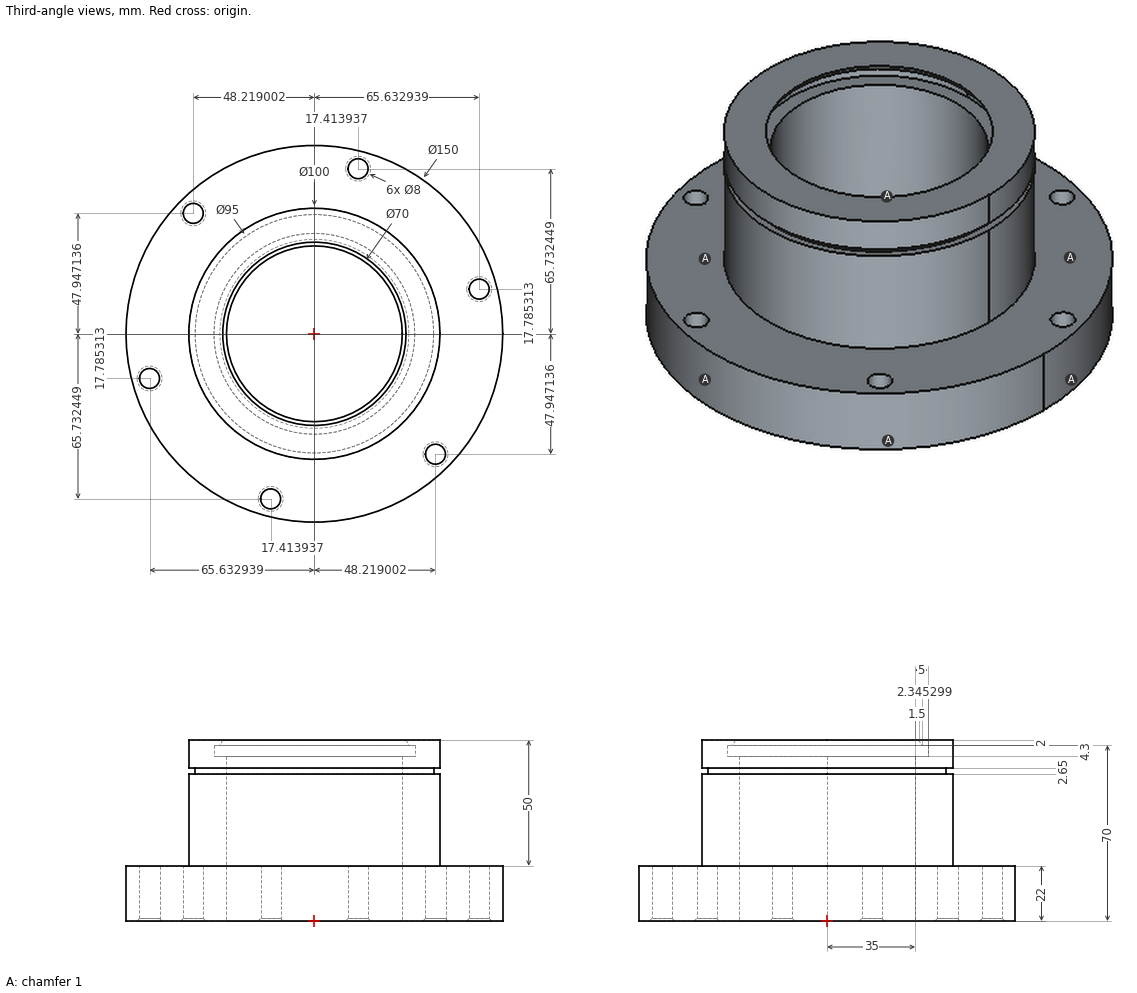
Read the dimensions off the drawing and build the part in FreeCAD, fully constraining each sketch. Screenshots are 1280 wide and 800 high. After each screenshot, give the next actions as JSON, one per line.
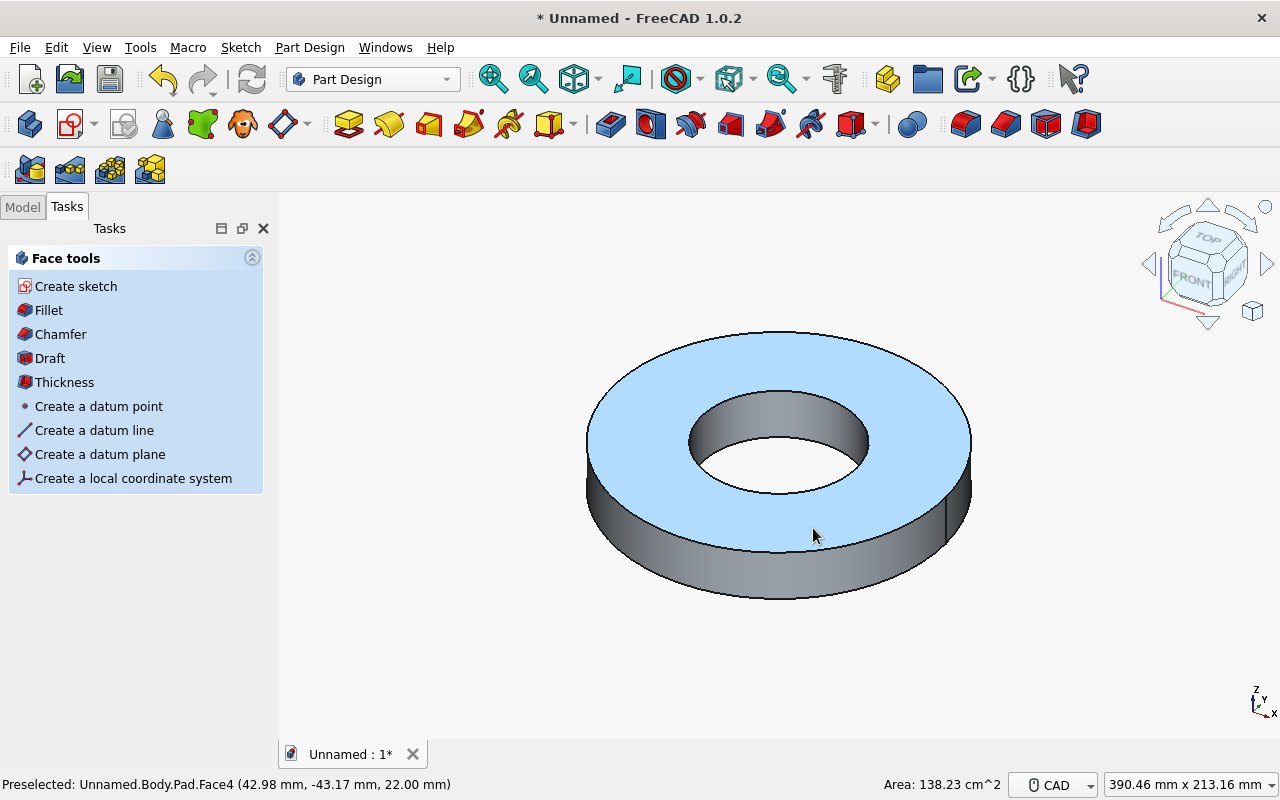
{"action": "left_click", "coordinate": [70, 124]}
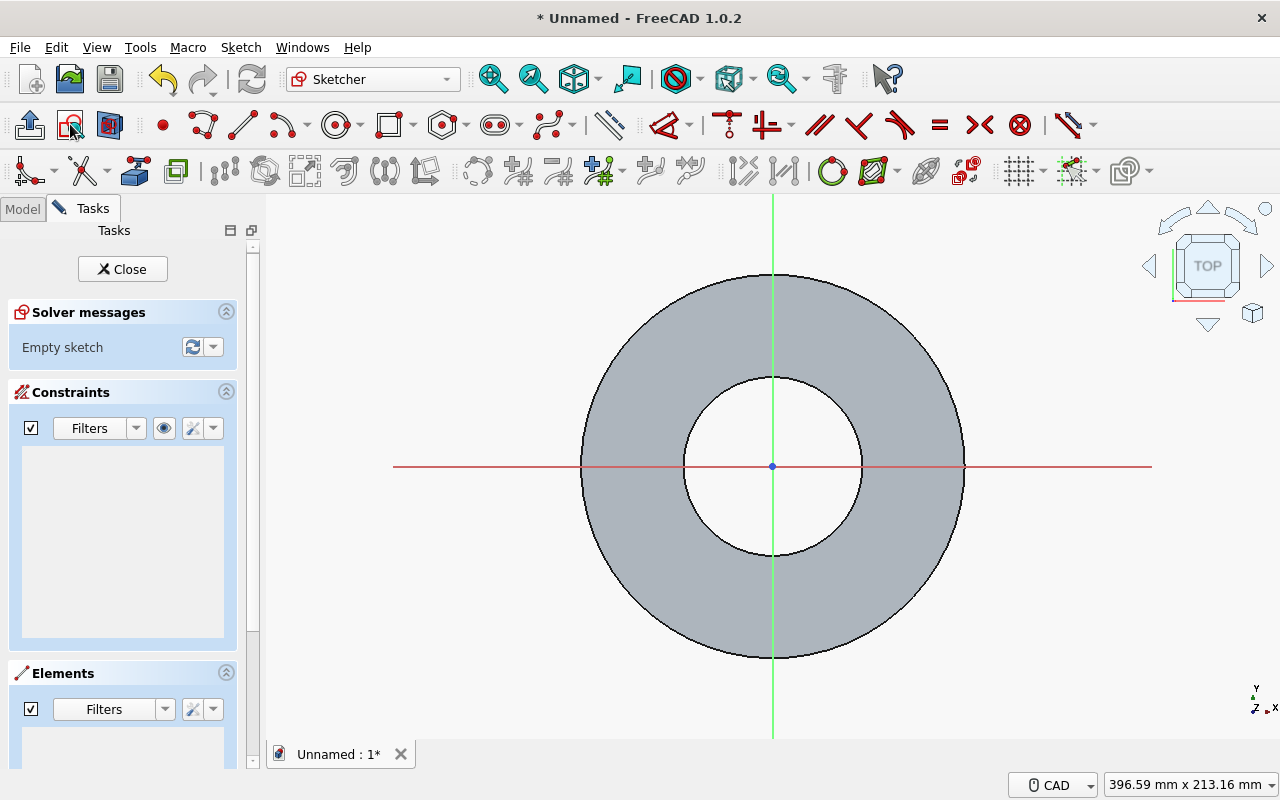
{"action": "left_click", "coordinate": [336, 126]}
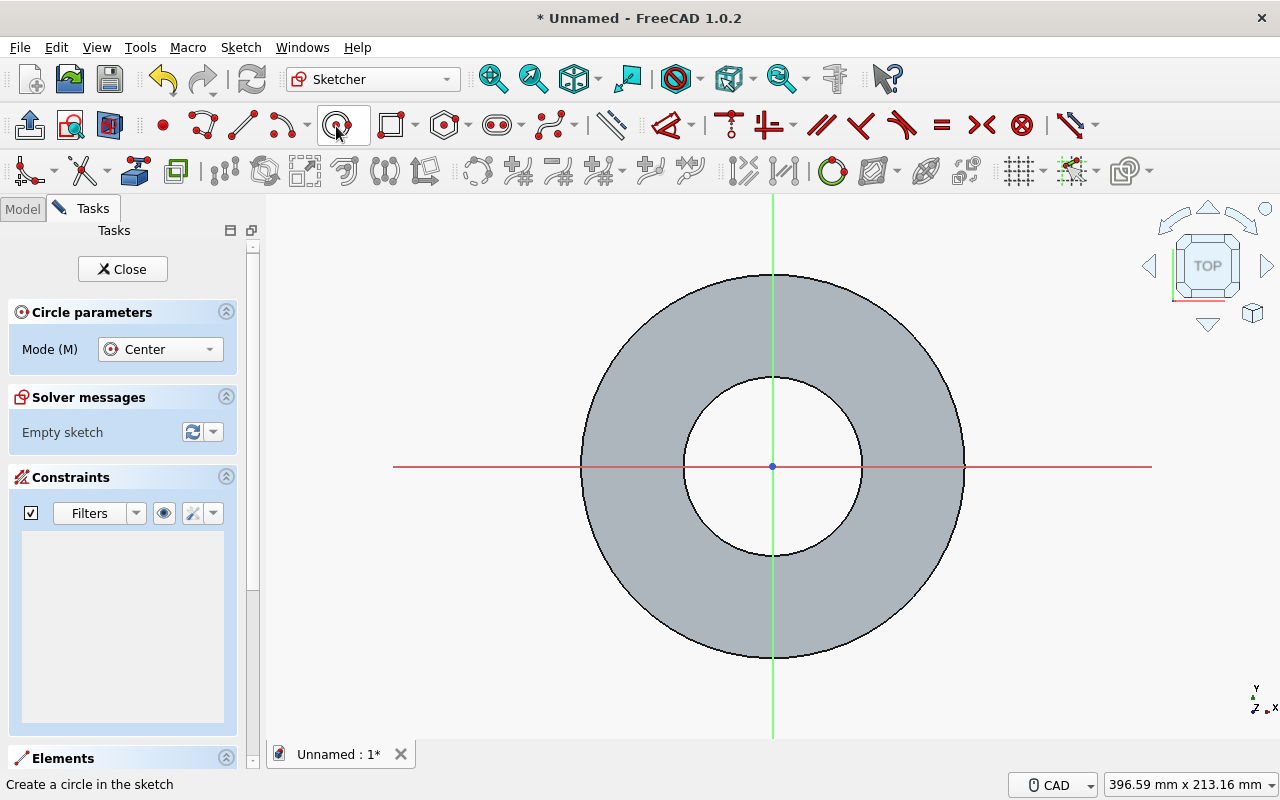
{"action": "left_click", "coordinate": [773, 466]}
{"action": "left_click", "coordinate": [863, 376]}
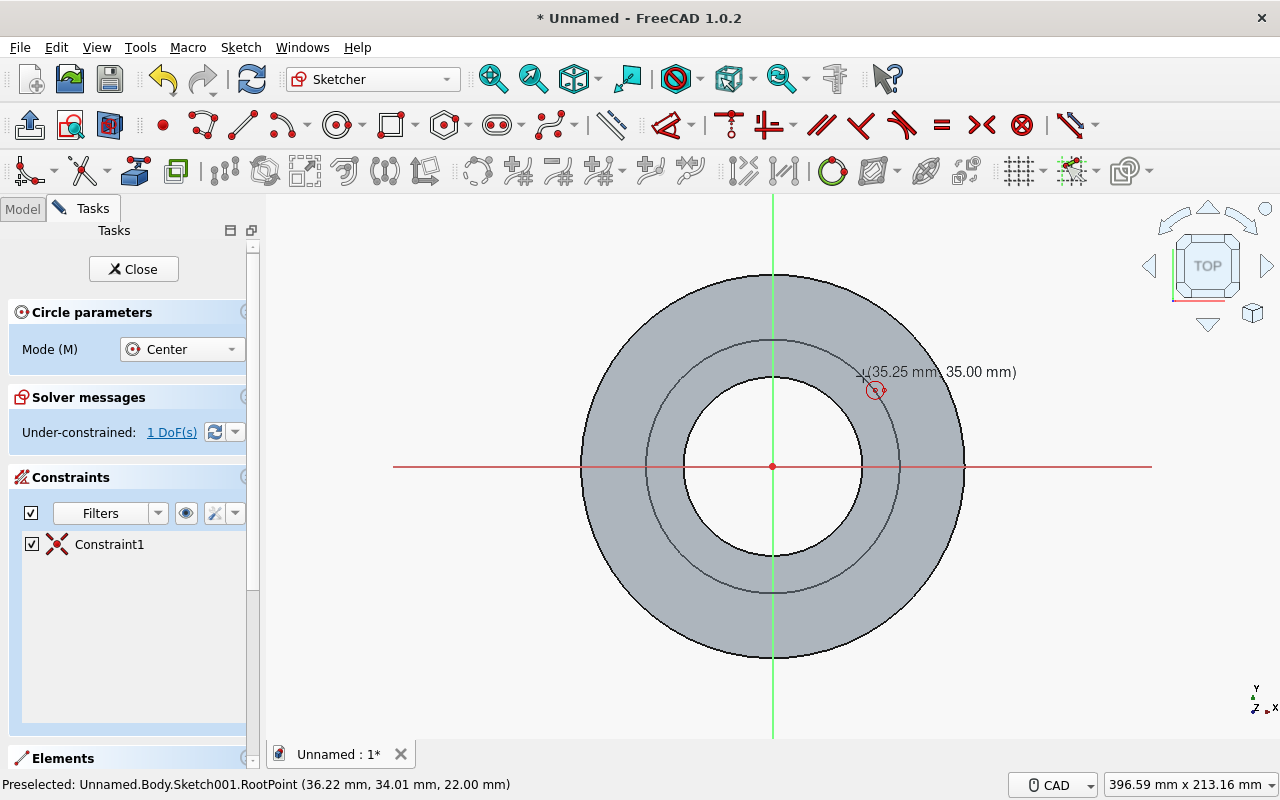
{"action": "left_click", "coordinate": [773, 466]}
{"action": "left_click", "coordinate": [836, 403]}
{"action": "key", "text": "Escape"}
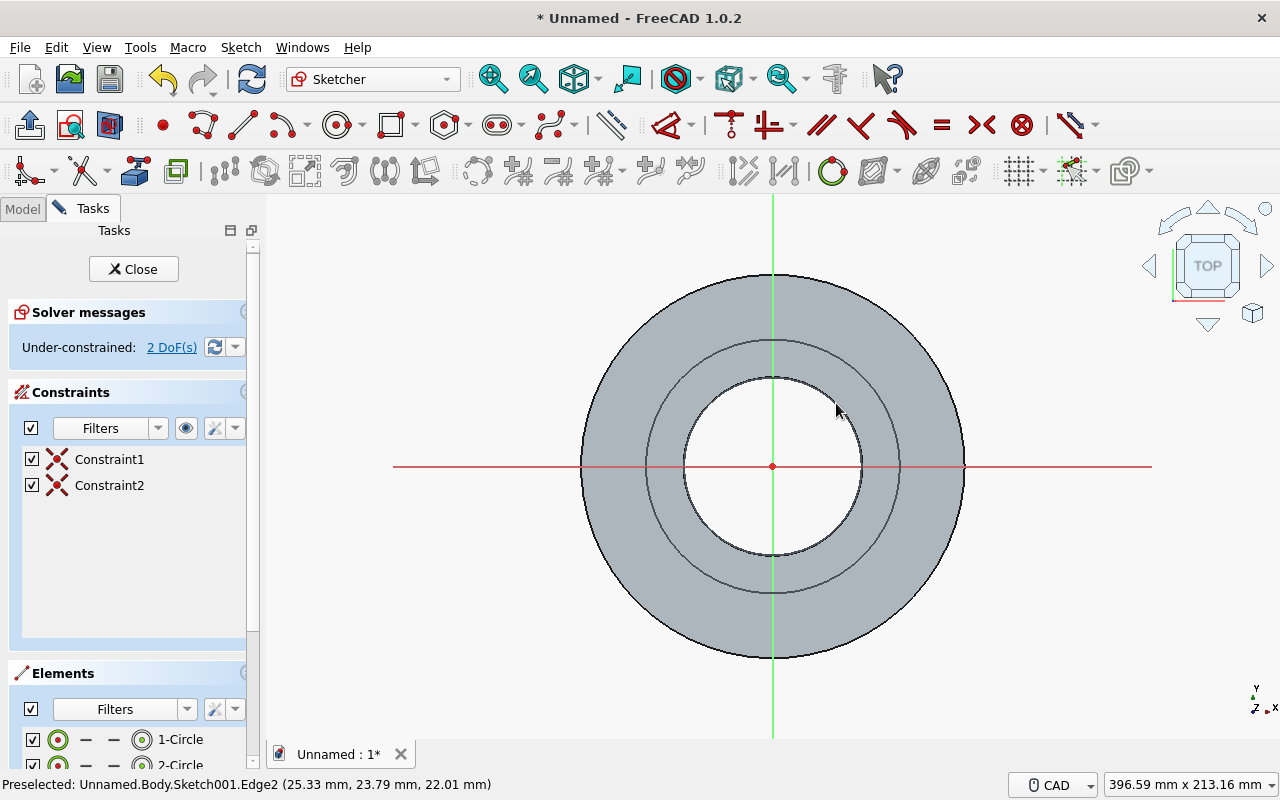
{"action": "key", "text": "d"}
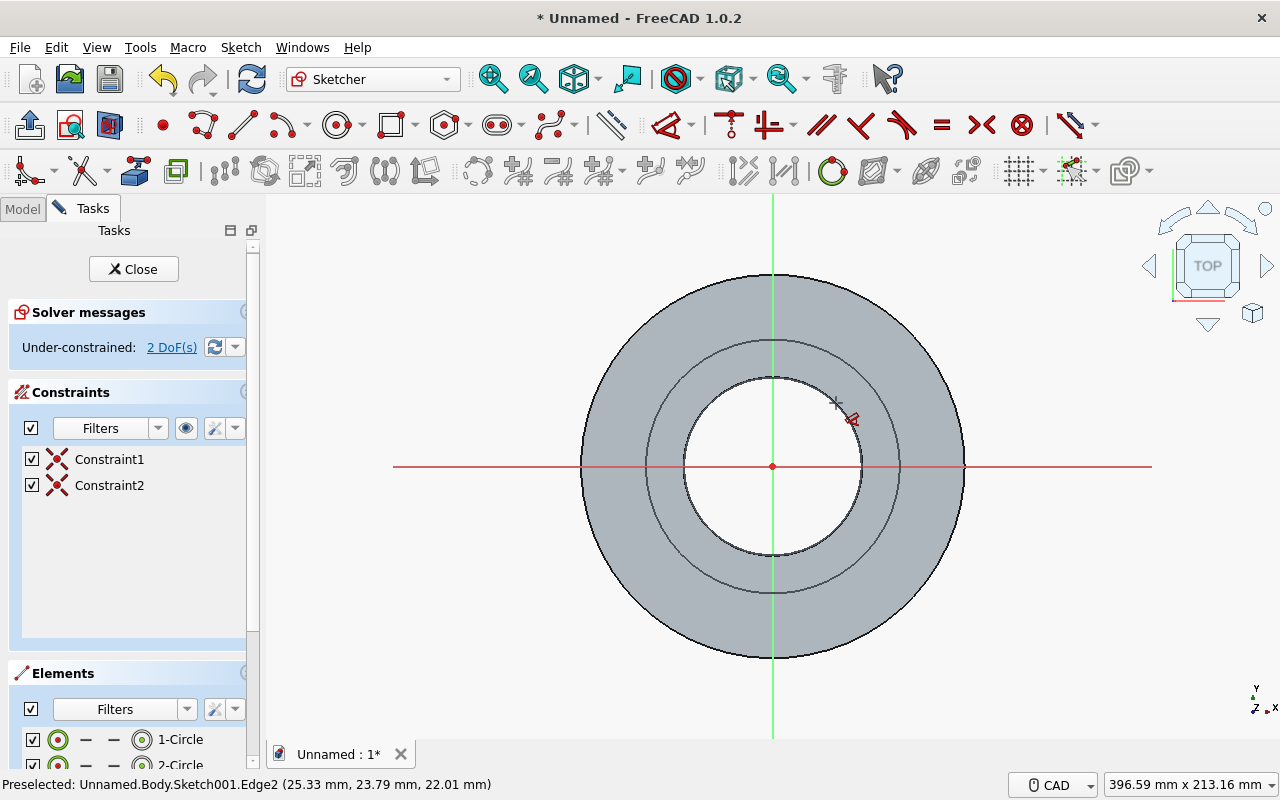
{"action": "left_click", "coordinate": [862, 376]}
{"action": "left_click", "coordinate": [884, 353]}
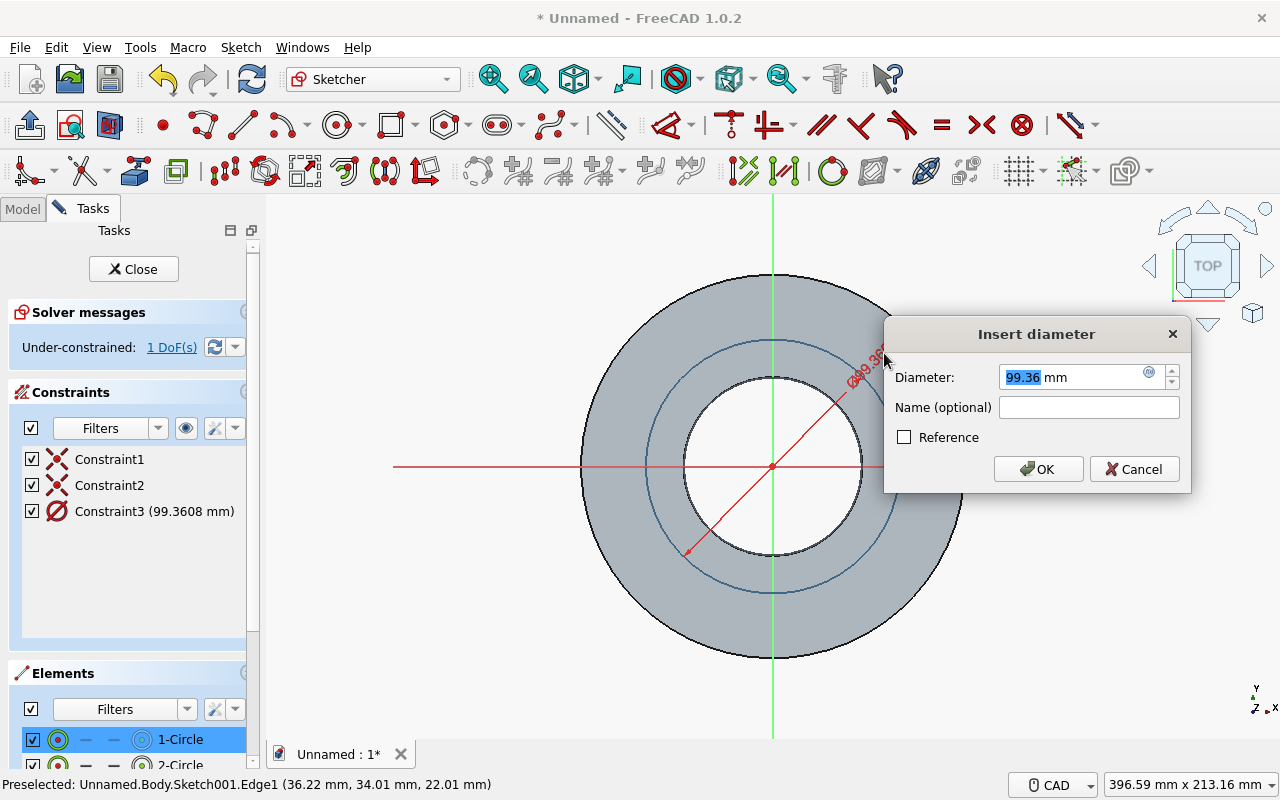
{"action": "type", "text": "100"}
{"action": "key", "text": "Return"}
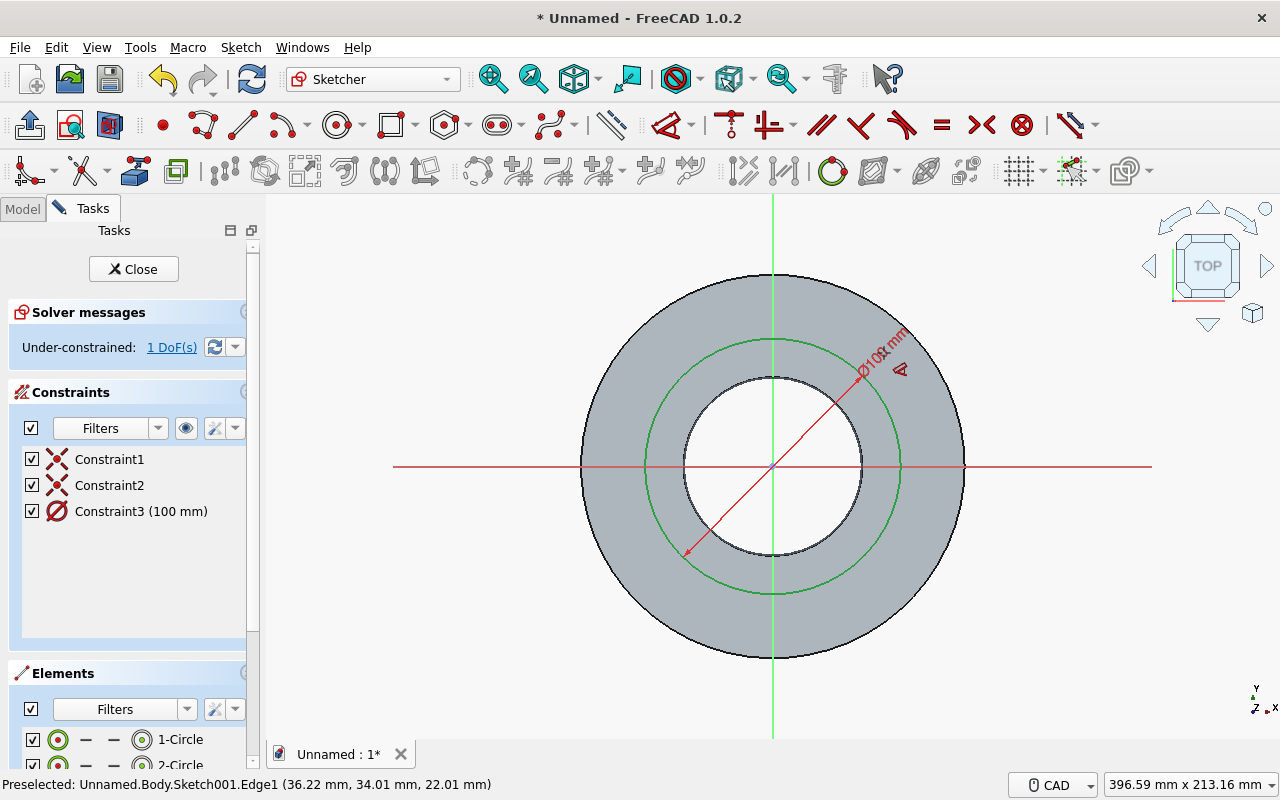
{"action": "left_click", "coordinate": [835, 403]}
{"action": "left_click", "coordinate": [910, 425]}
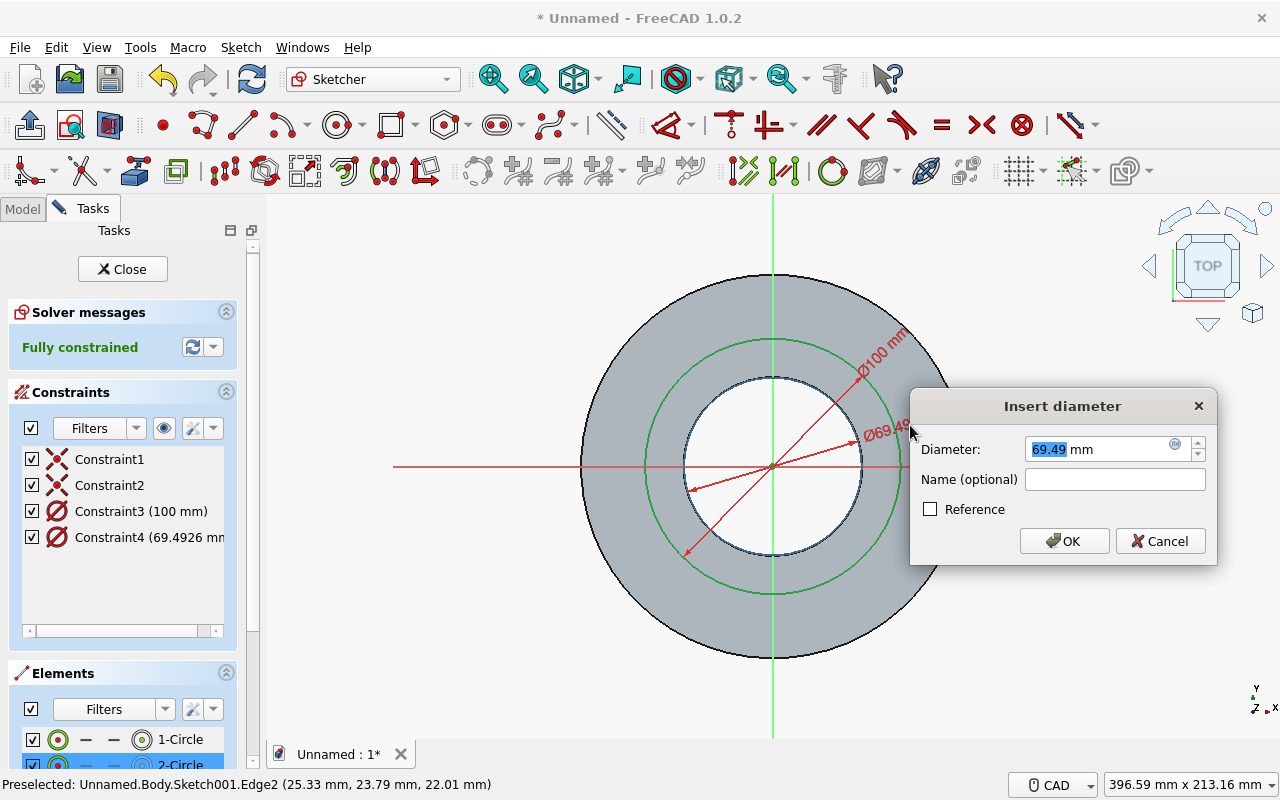
{"action": "type", "text": "70"}
{"action": "key", "text": "Return"}
{"action": "key", "text": "Escape"}